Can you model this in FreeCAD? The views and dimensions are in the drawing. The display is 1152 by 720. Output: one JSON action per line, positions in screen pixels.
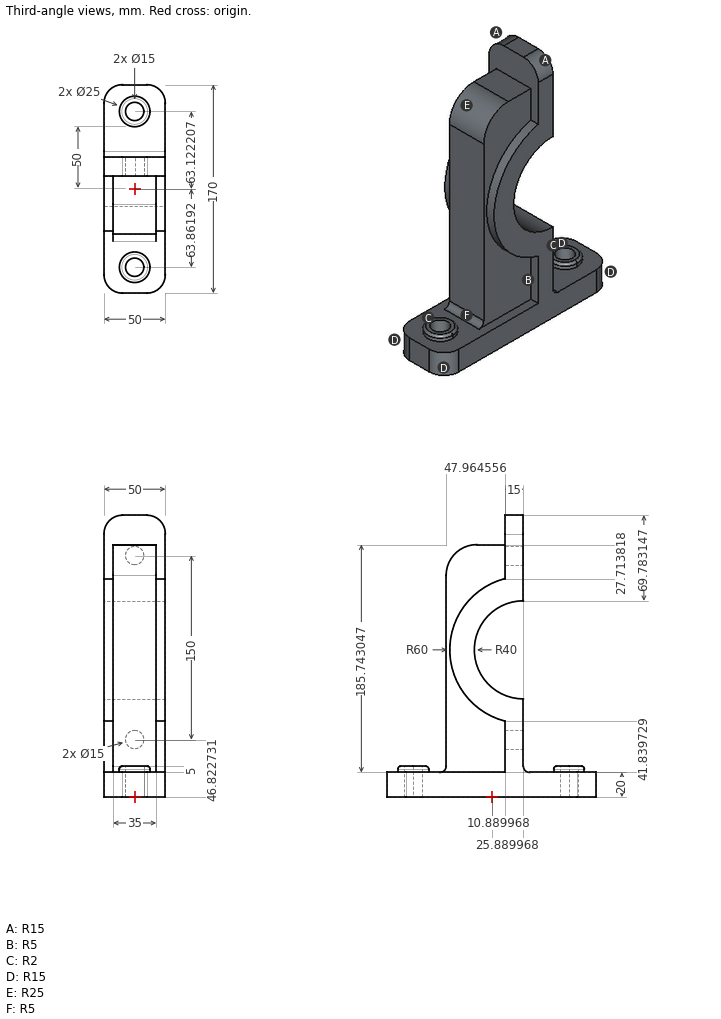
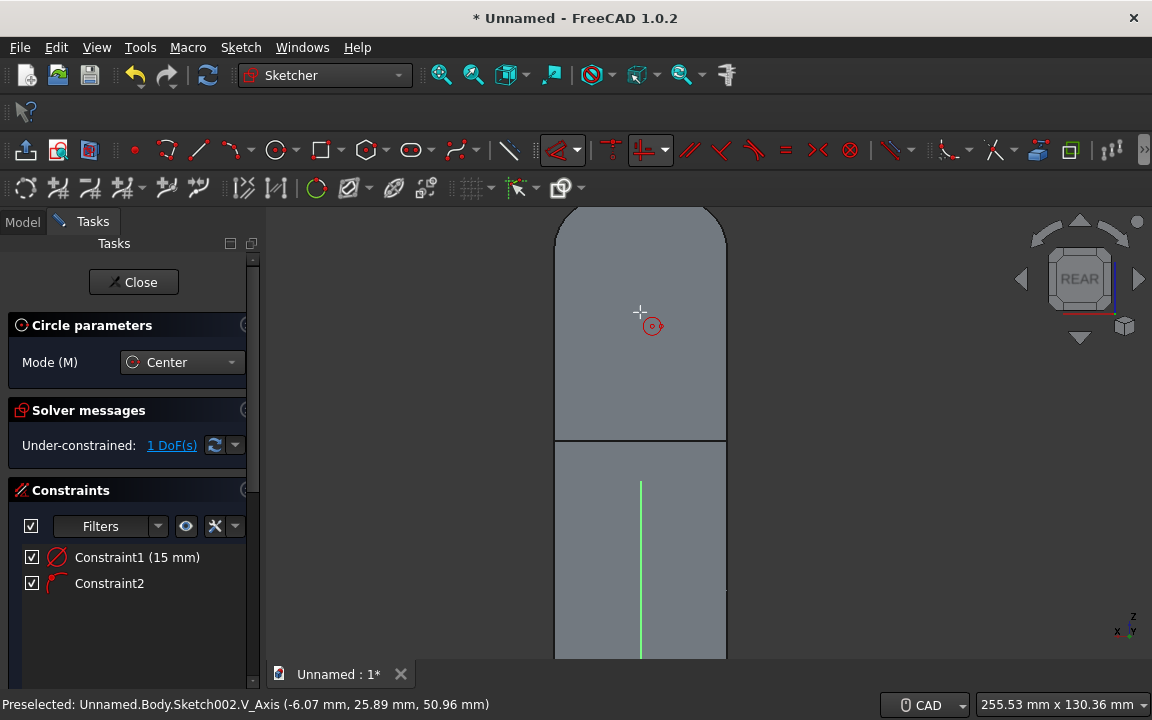
{"action": "left_click", "coordinate": [641, 313]}
{"action": "mouse_move", "coordinate": [659, 294]}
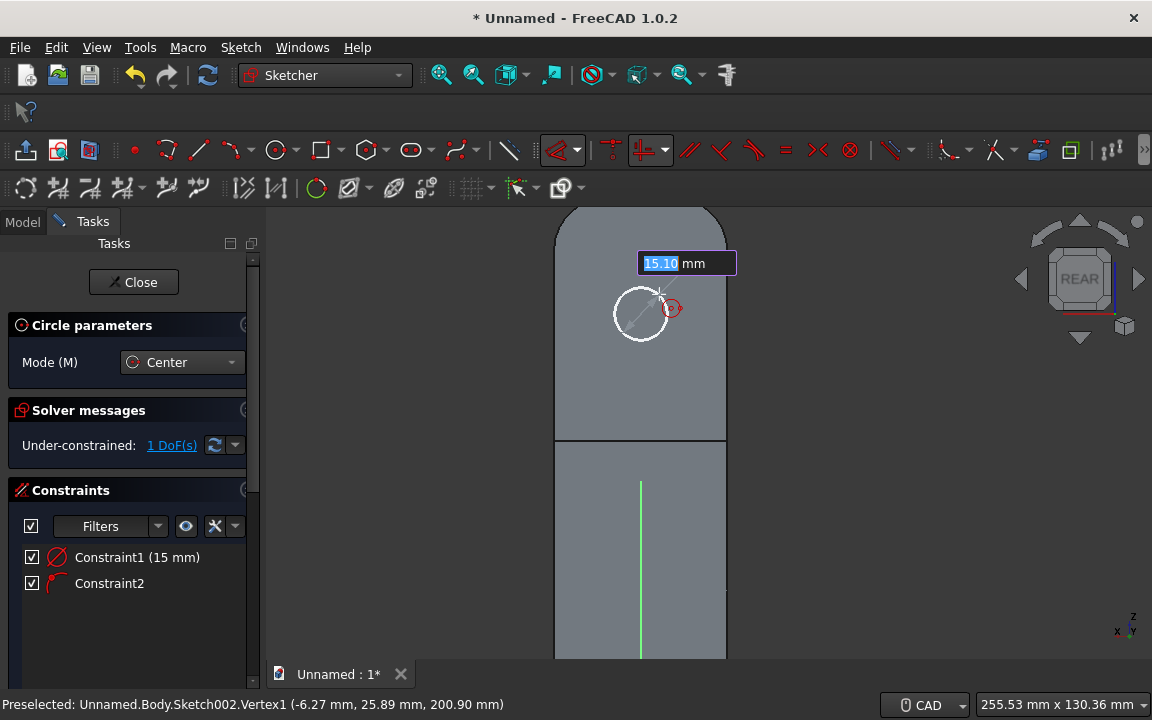
{"action": "type", "text": "15"}
{"action": "key", "text": "Return"}
{"action": "key", "text": "Escape"}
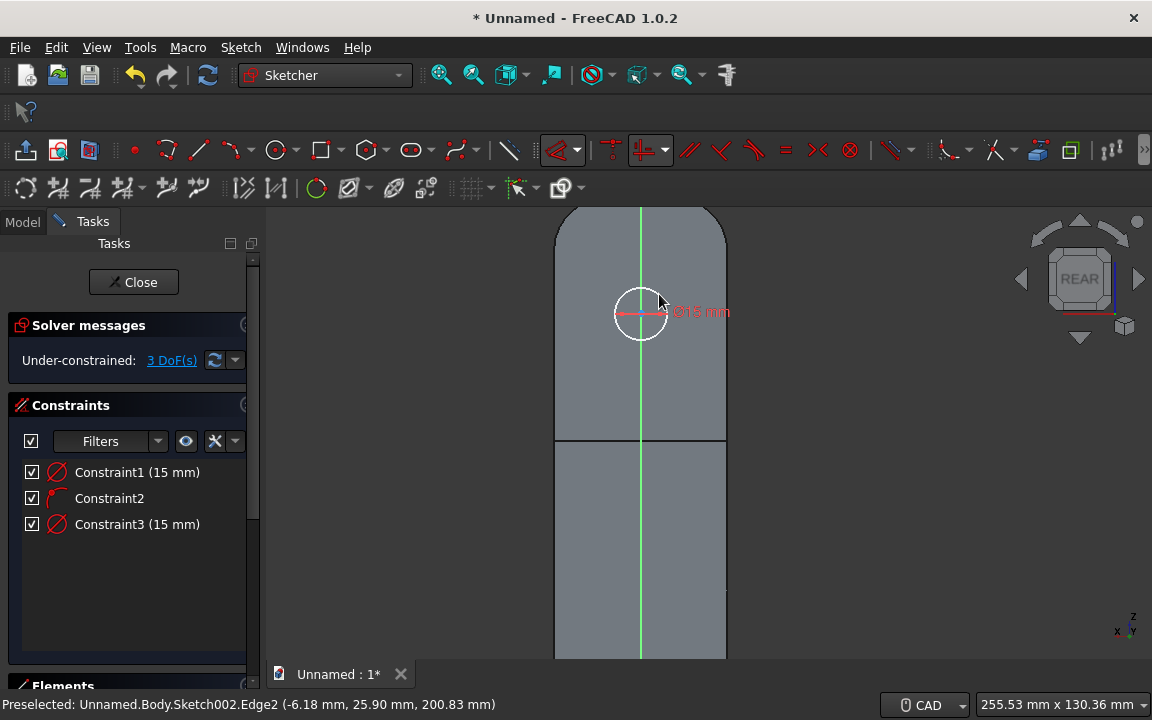
{"action": "left_click", "coordinate": [641, 314]}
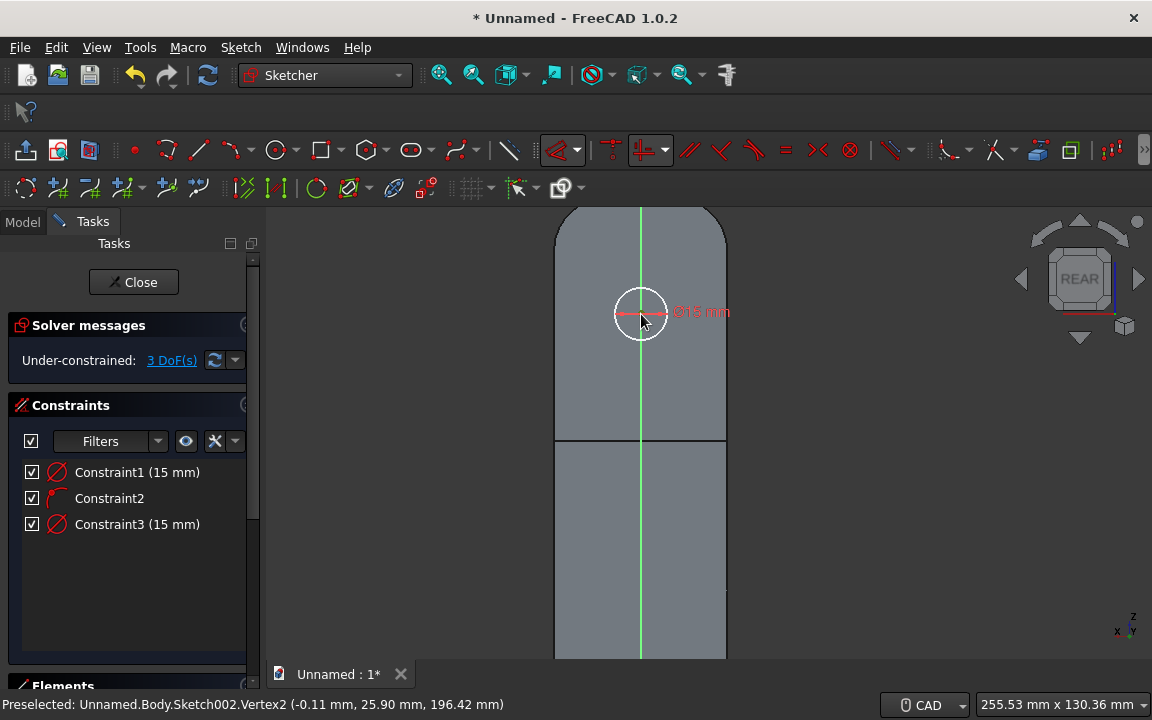
{"action": "left_click", "coordinate": [641, 603]}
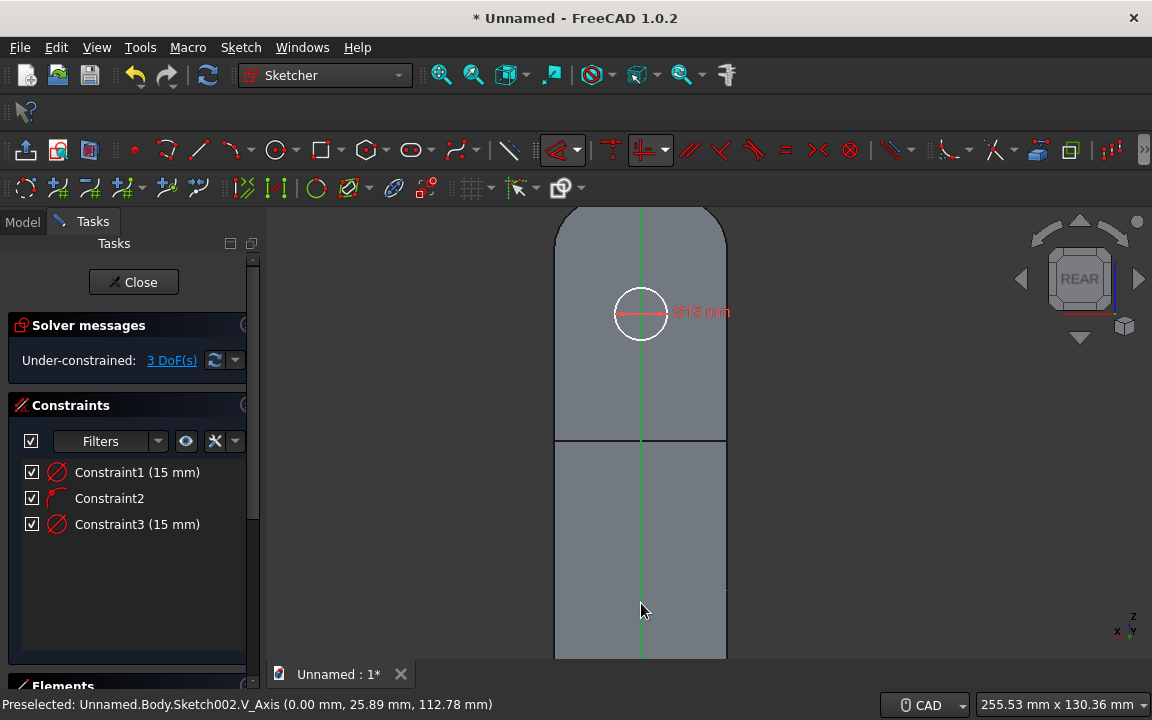
{"action": "key", "text": "c"}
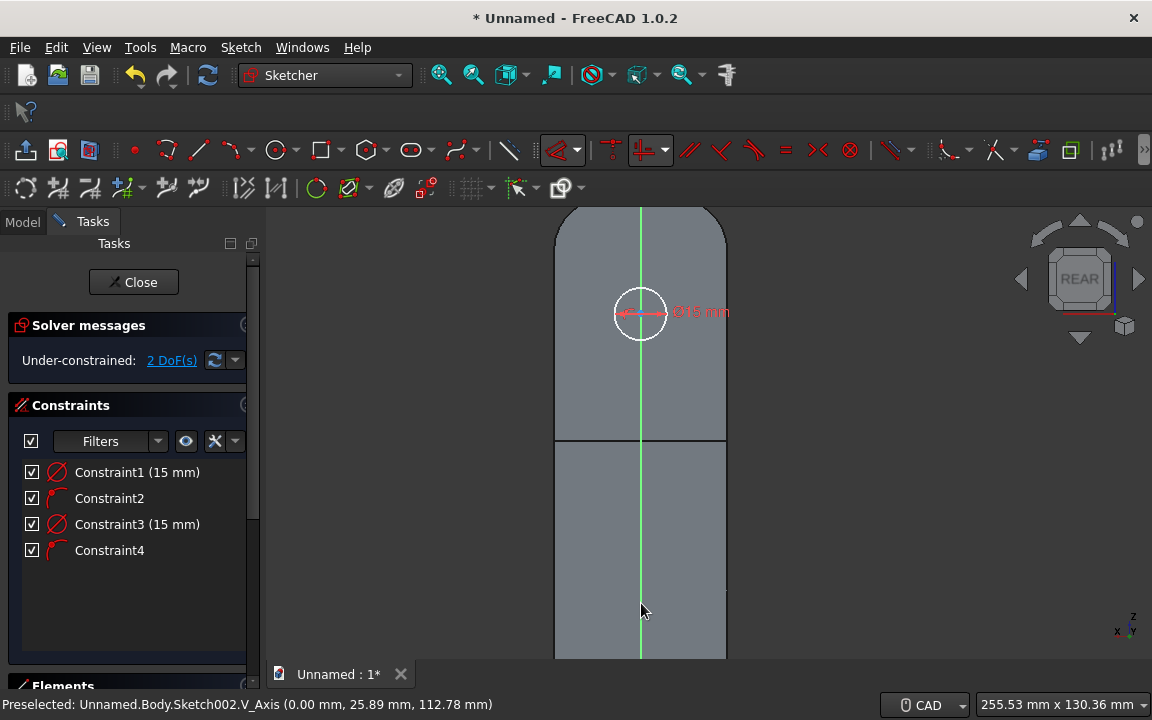
{"action": "scroll", "coordinate": [640, 312], "scroll_direction": "down", "scroll_amount": 5}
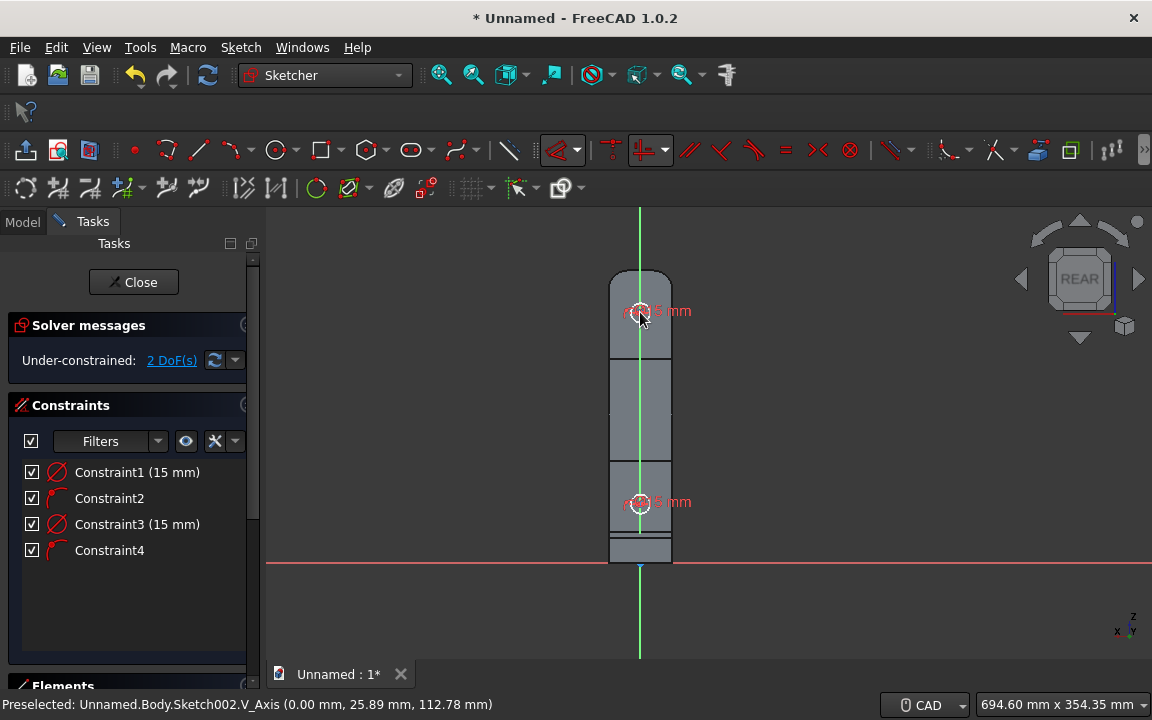
{"action": "left_click", "coordinate": [640, 504]}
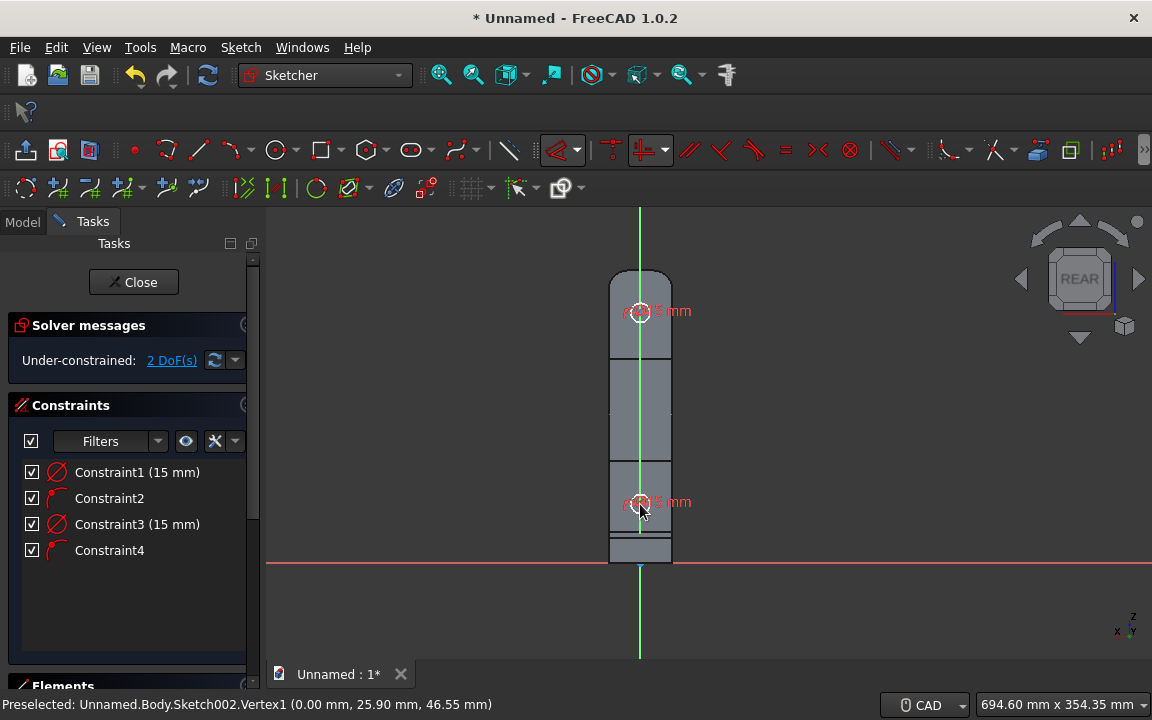
{"action": "left_click", "coordinate": [640, 313]}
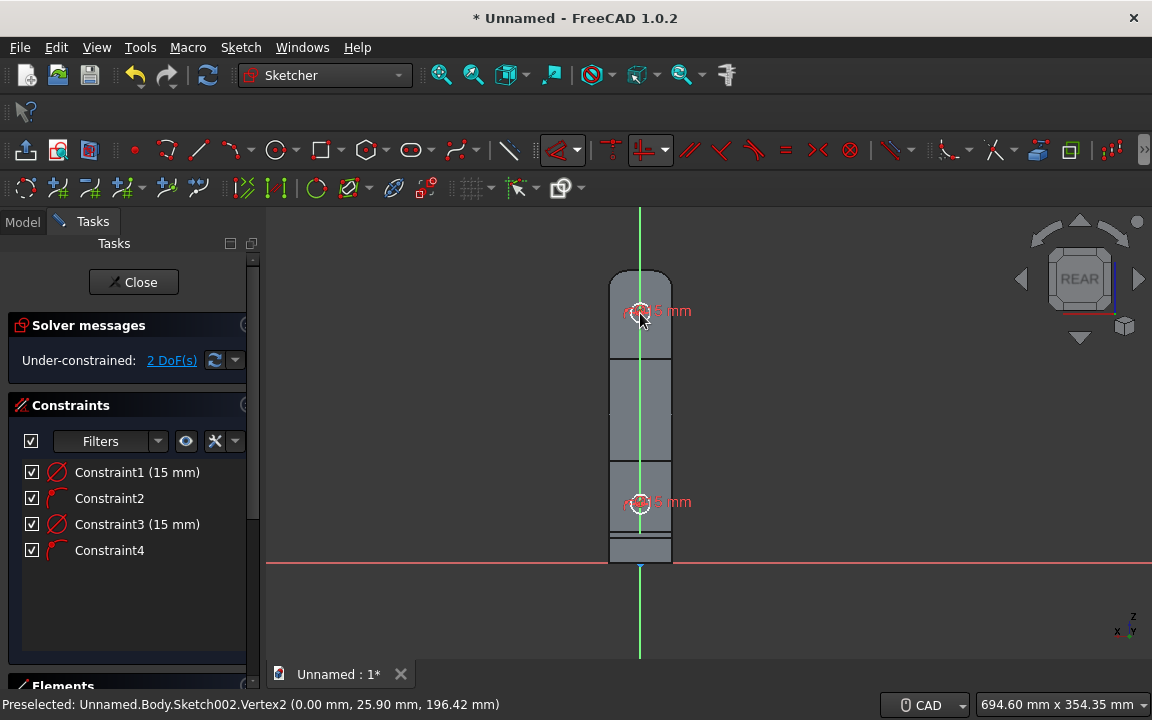
{"action": "key", "text": "i"}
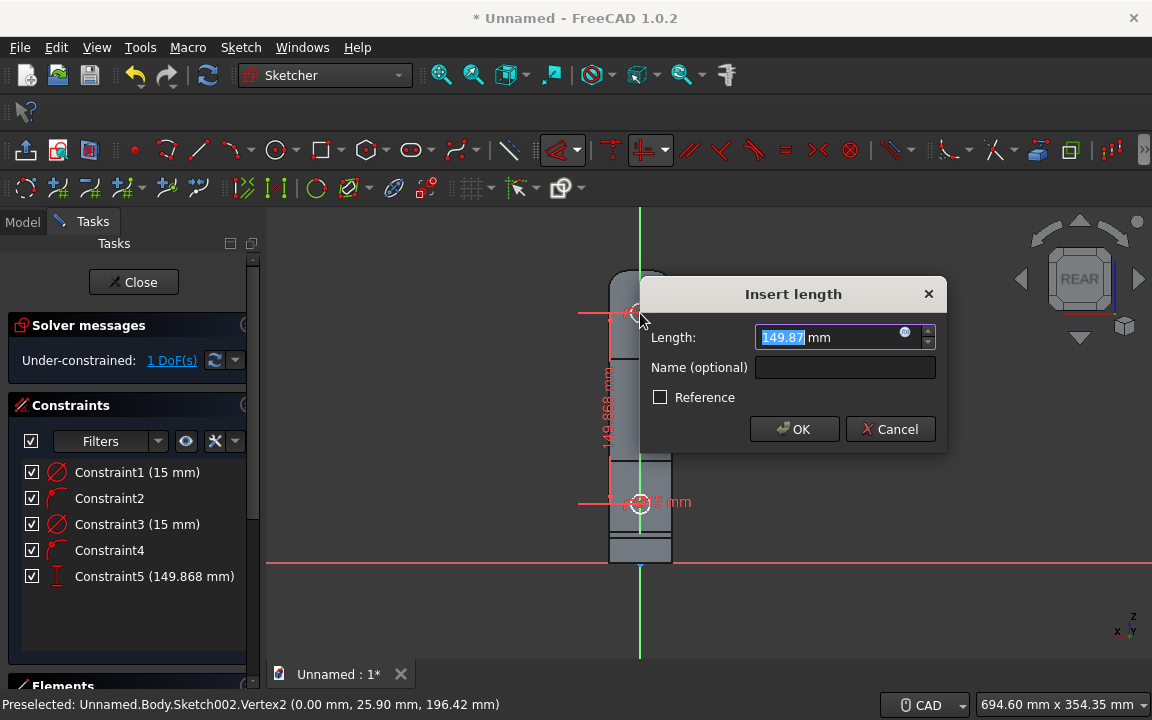
{"action": "type", "text": "150"}
{"action": "key", "text": "Return"}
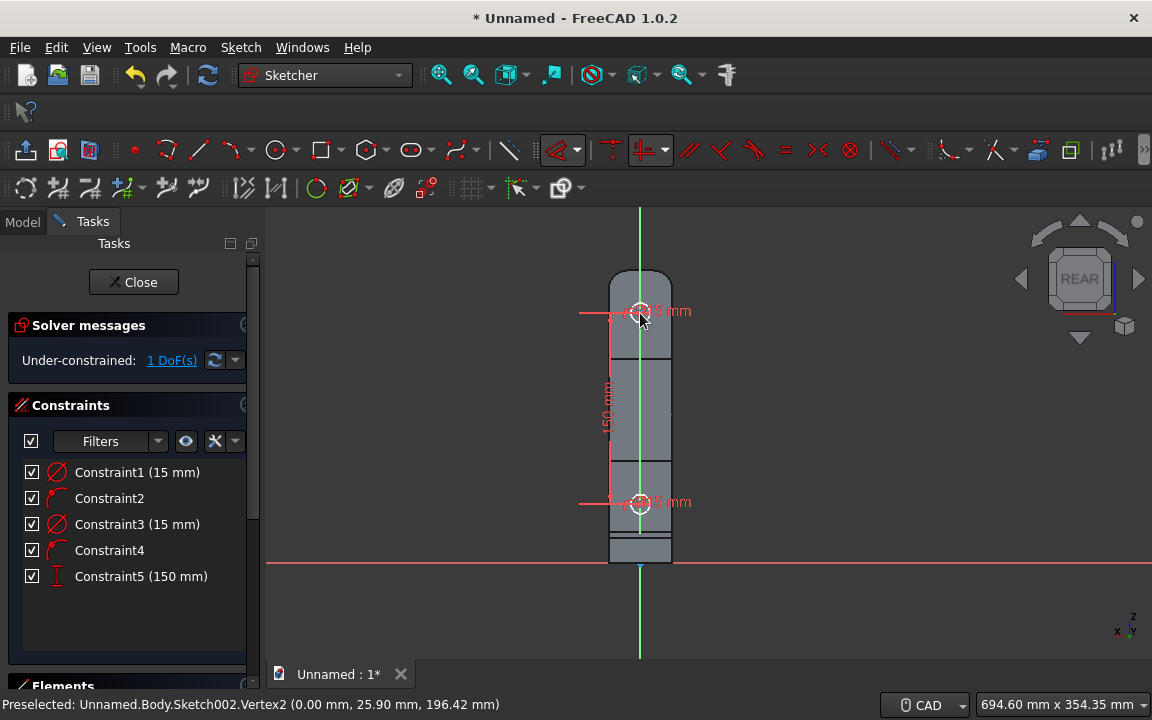
{"action": "left_click", "coordinate": [640, 504]}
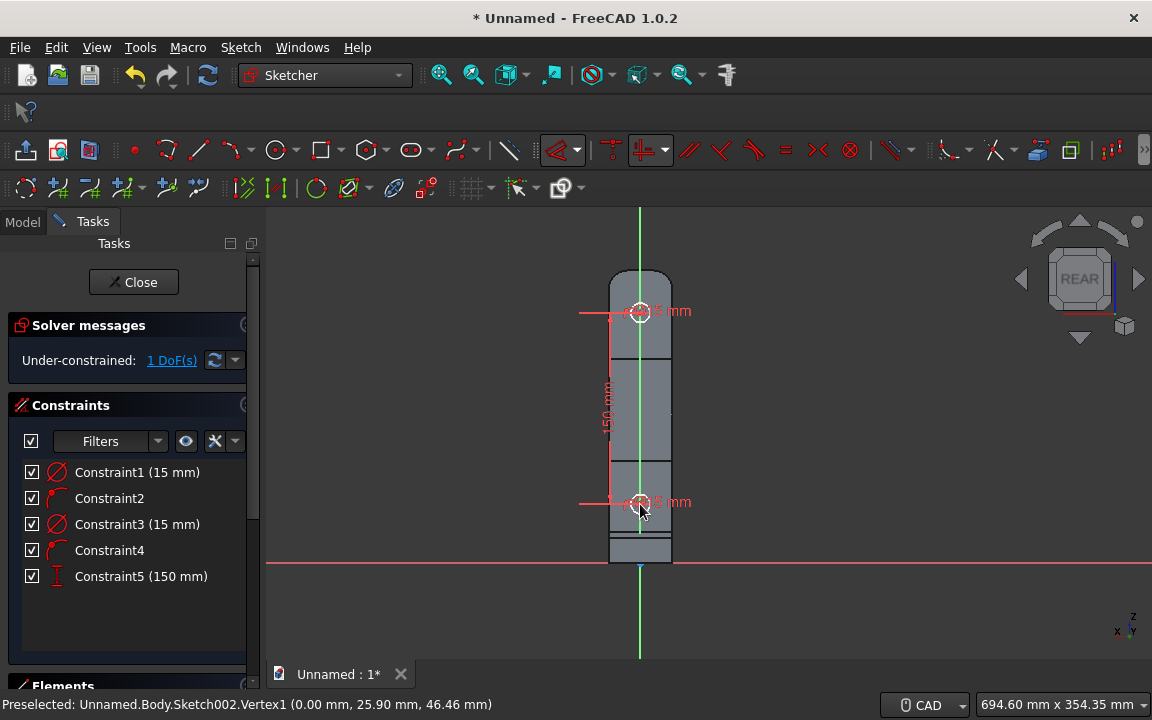
{"action": "key", "text": "i"}